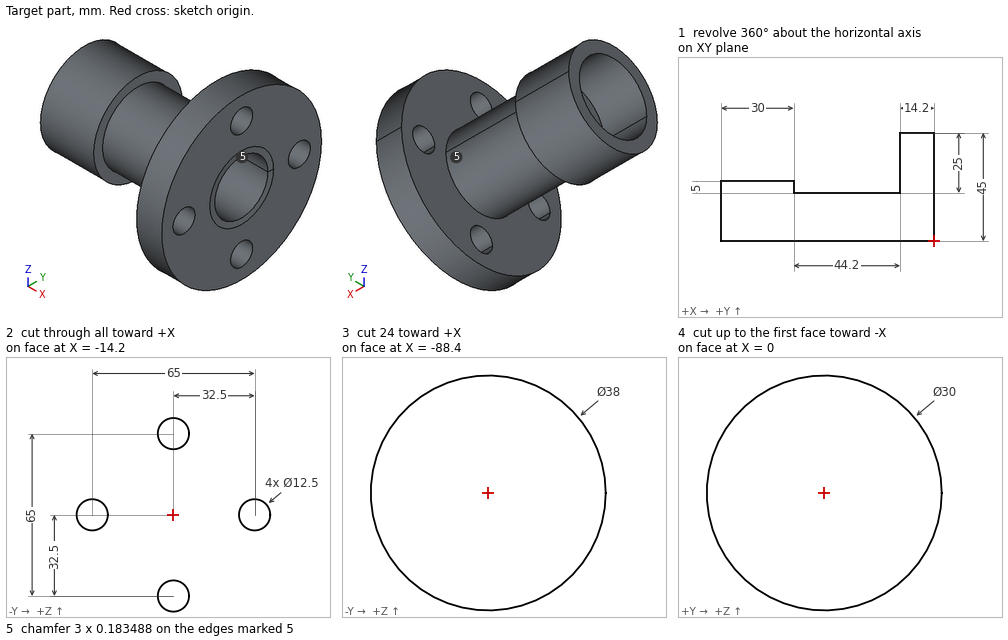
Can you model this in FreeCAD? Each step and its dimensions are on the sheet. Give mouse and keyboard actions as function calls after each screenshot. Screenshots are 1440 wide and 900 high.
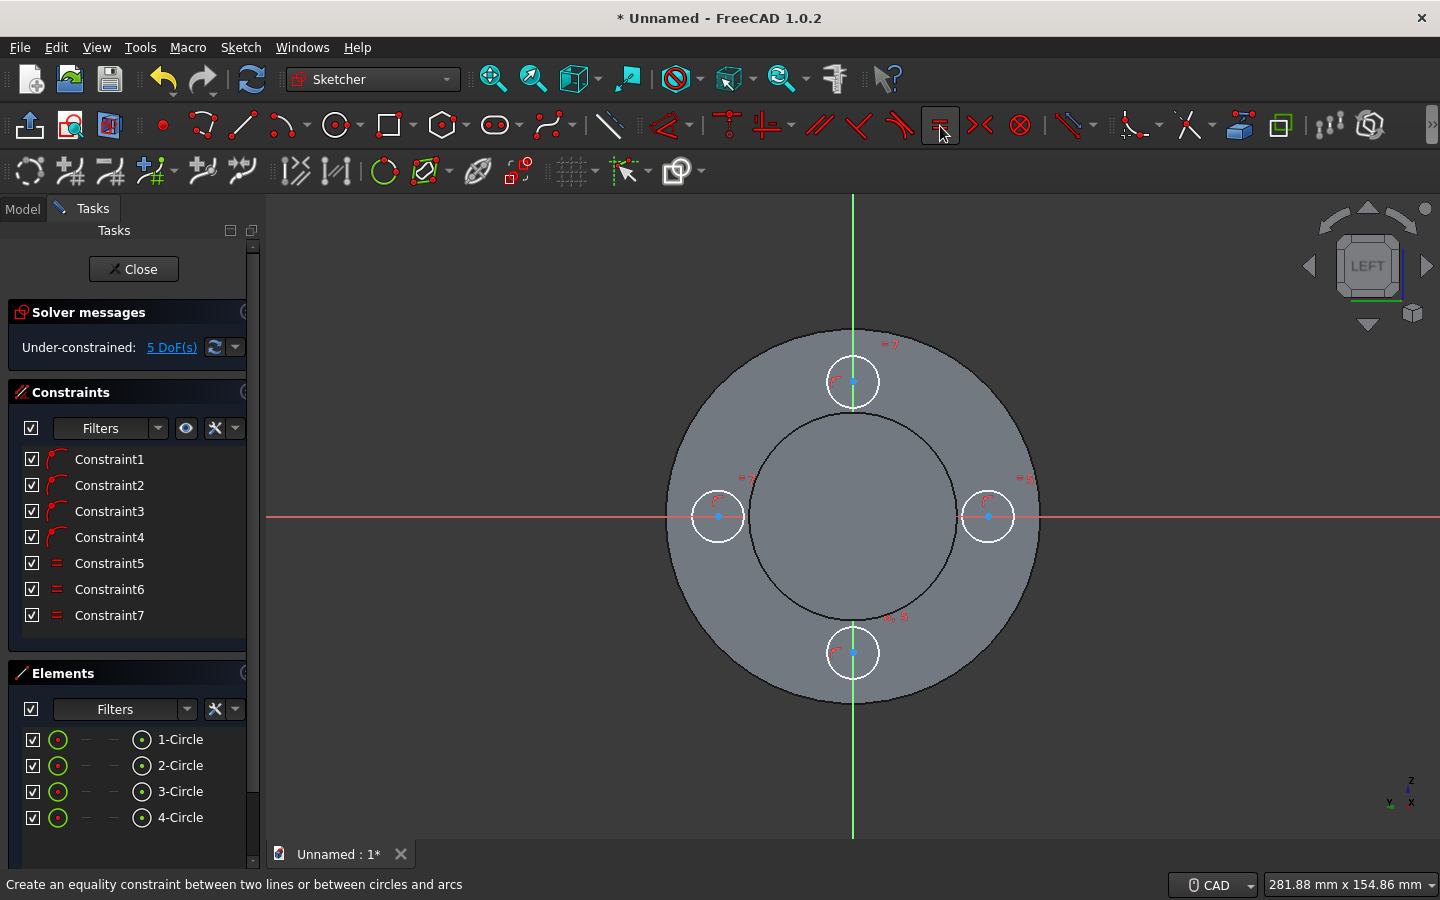
key(d)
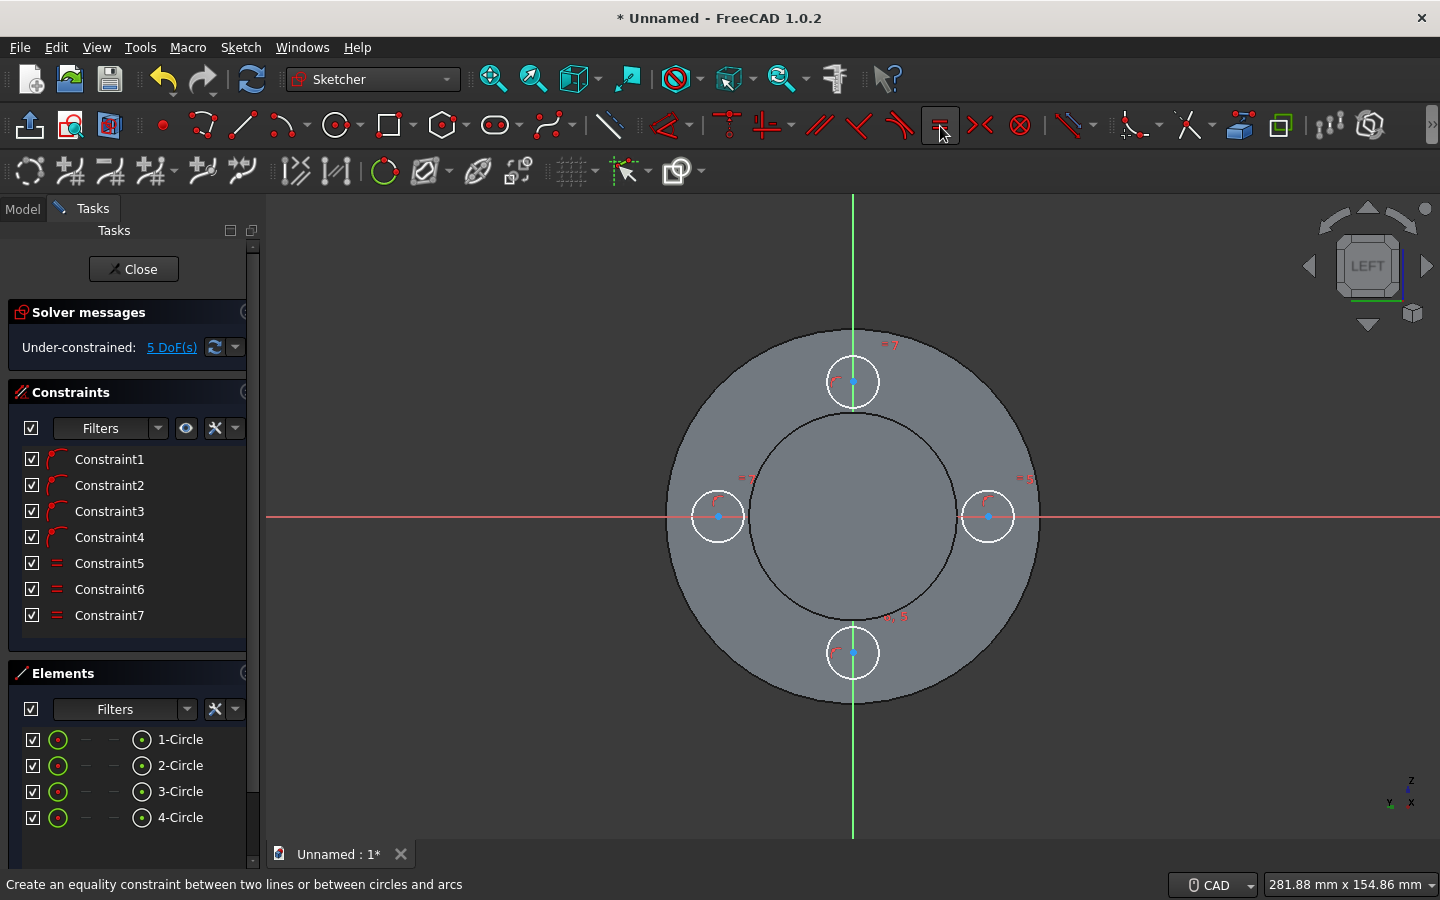
click(1006, 498)
click(1028, 475)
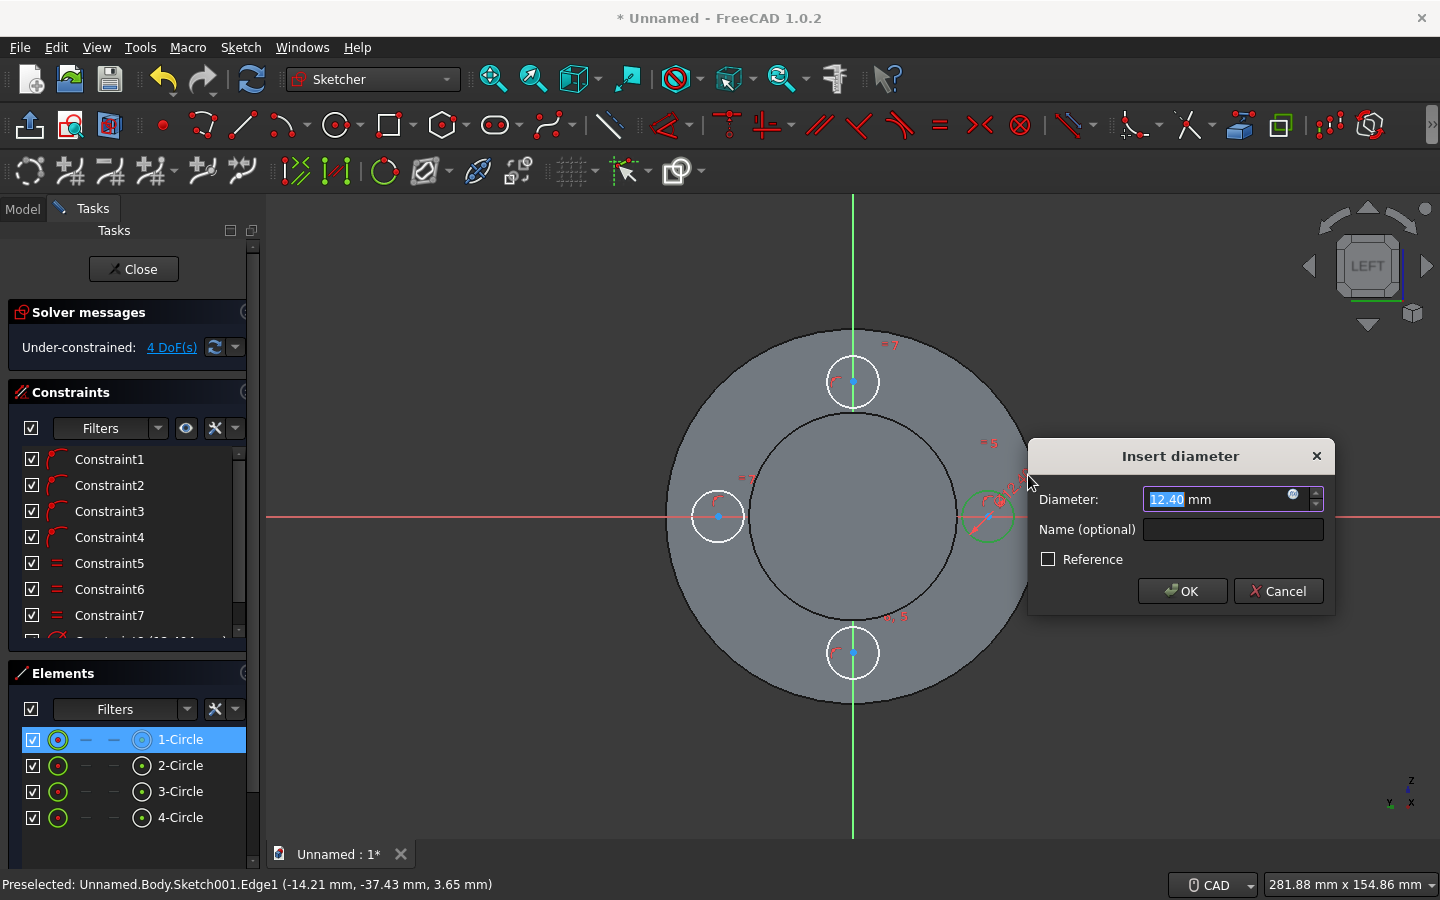
text(12.5)
key(Return)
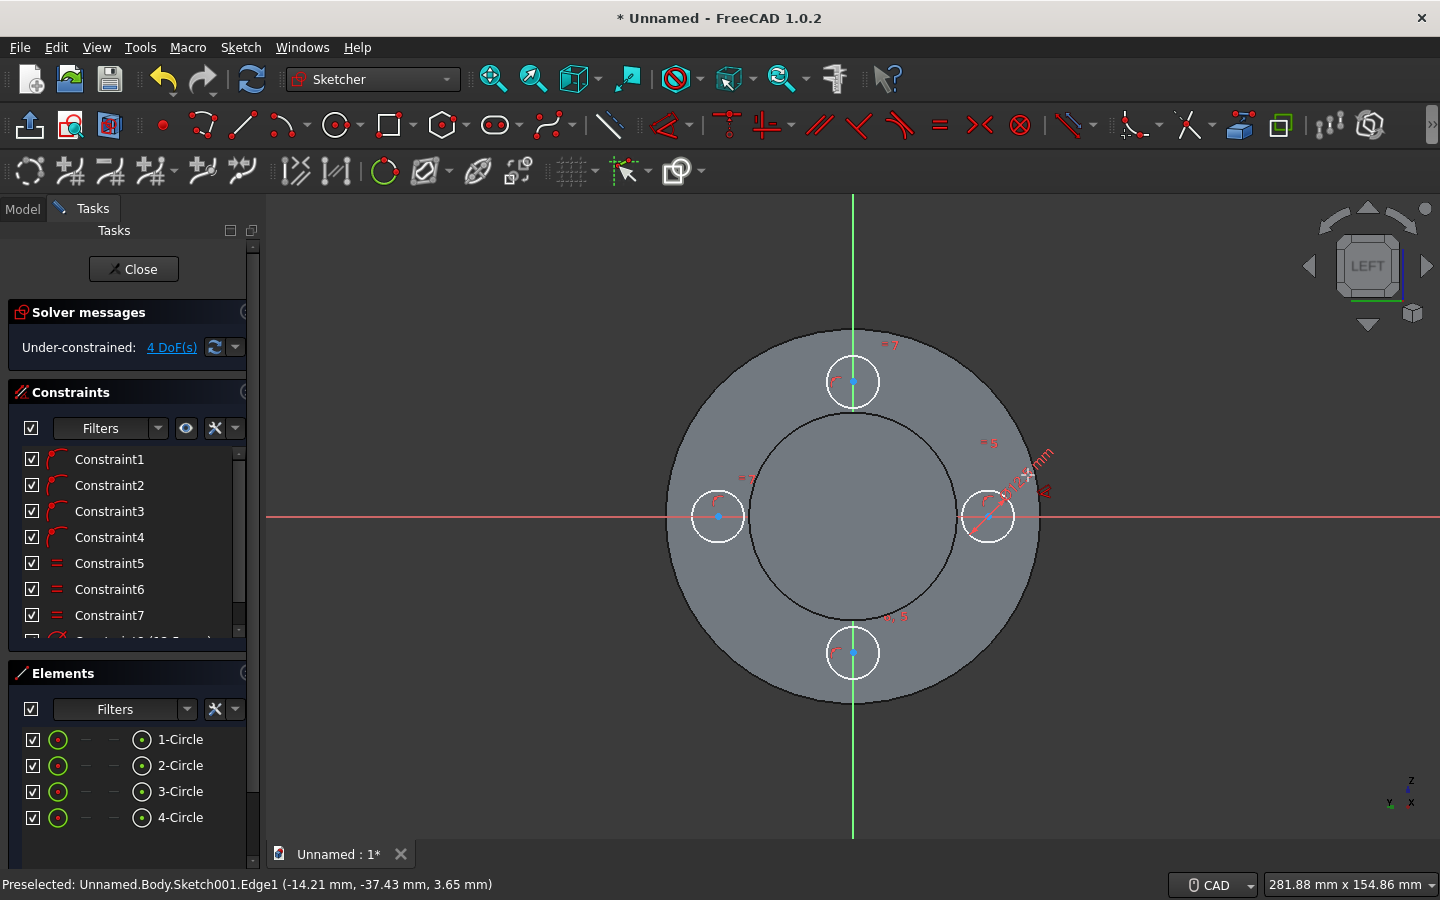
click(988, 516)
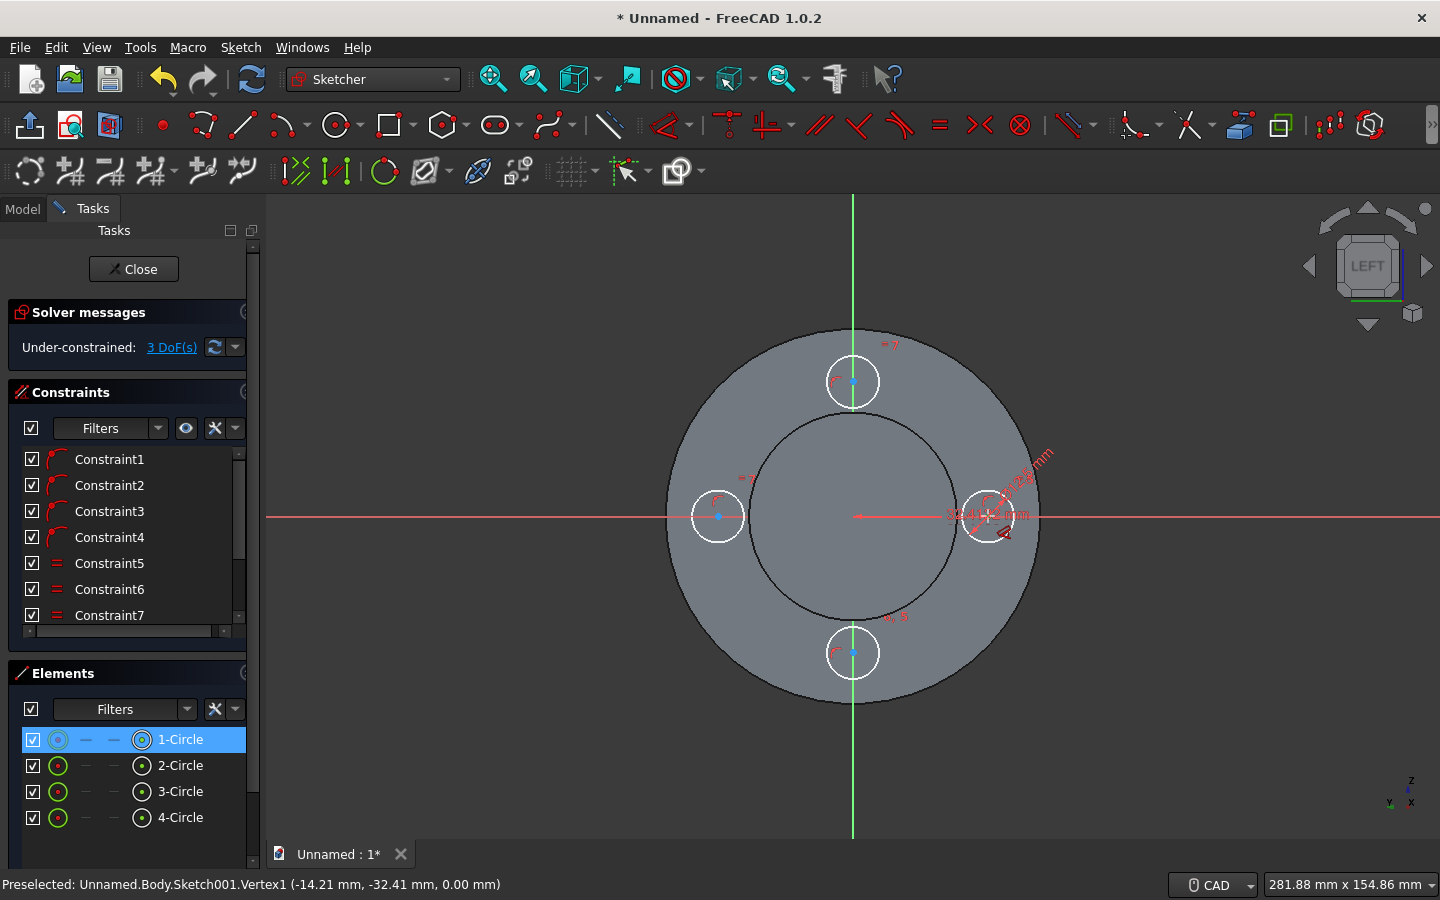
click(718, 516)
click(791, 550)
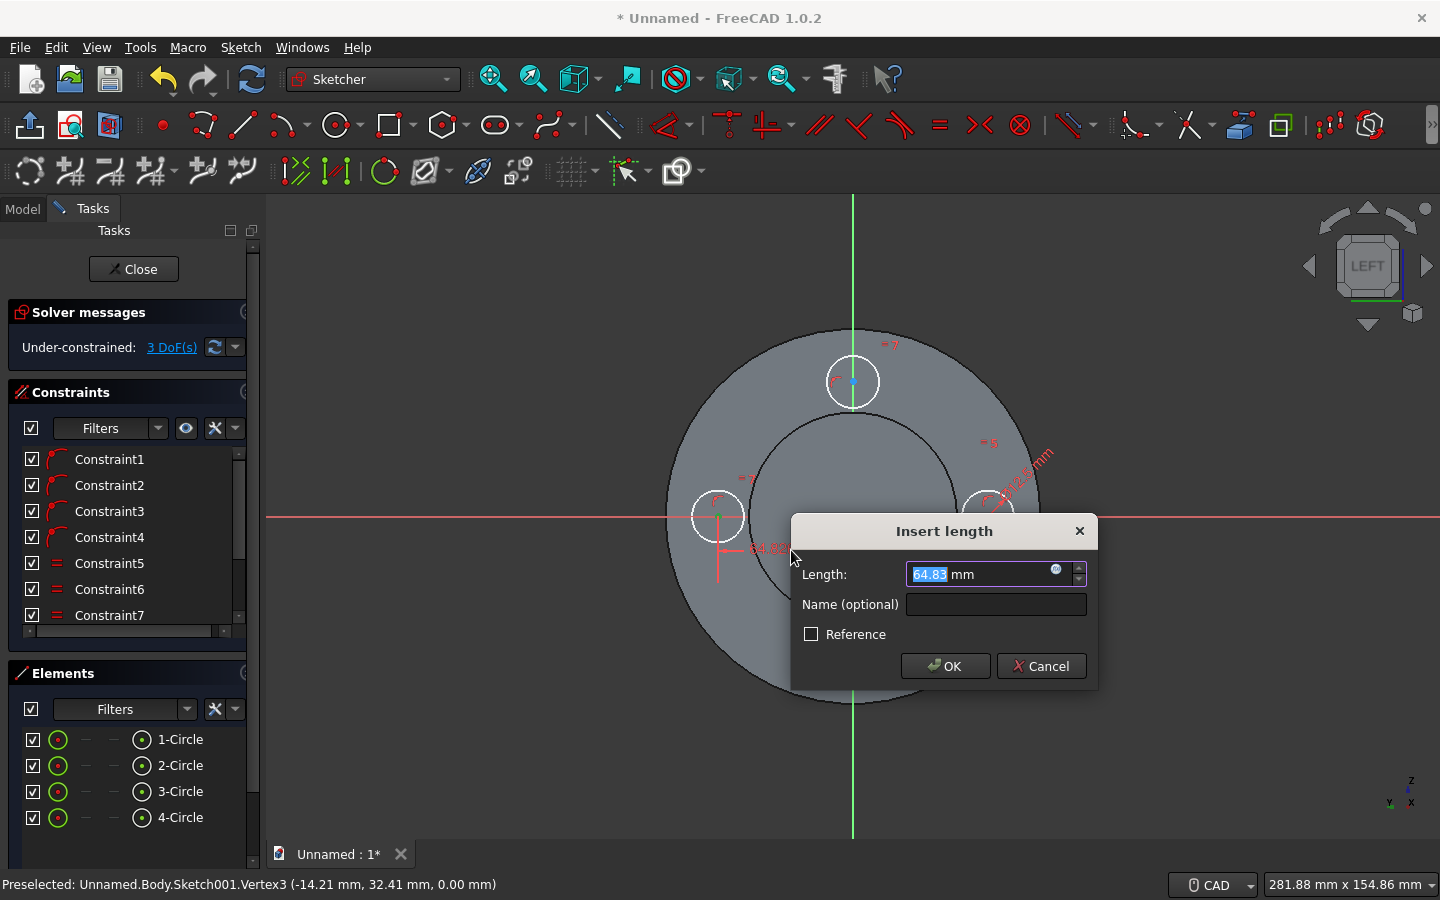
text(65)
key(Return)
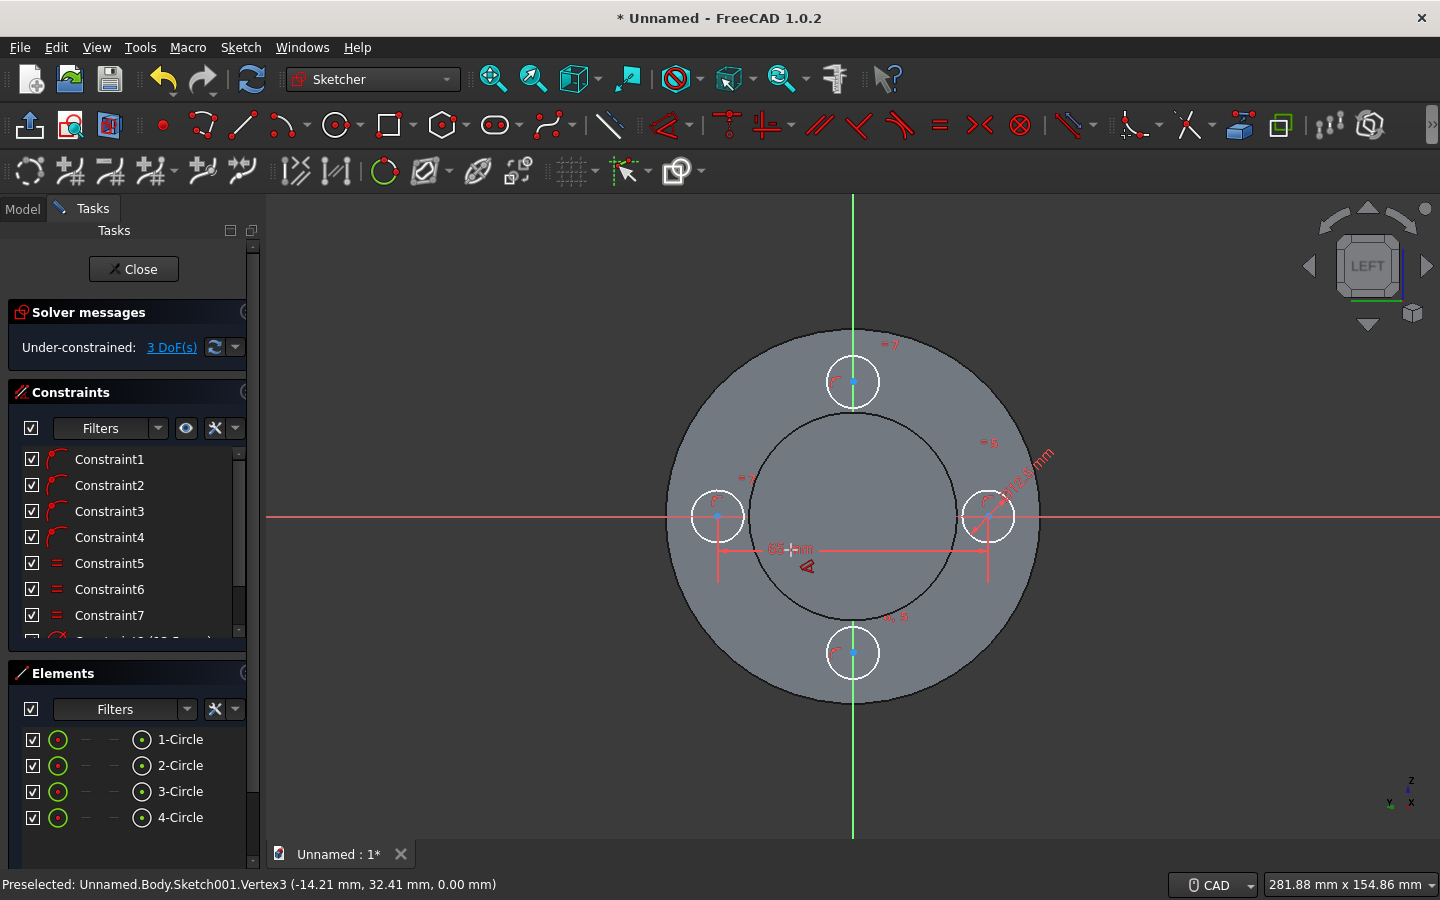
click(853, 653)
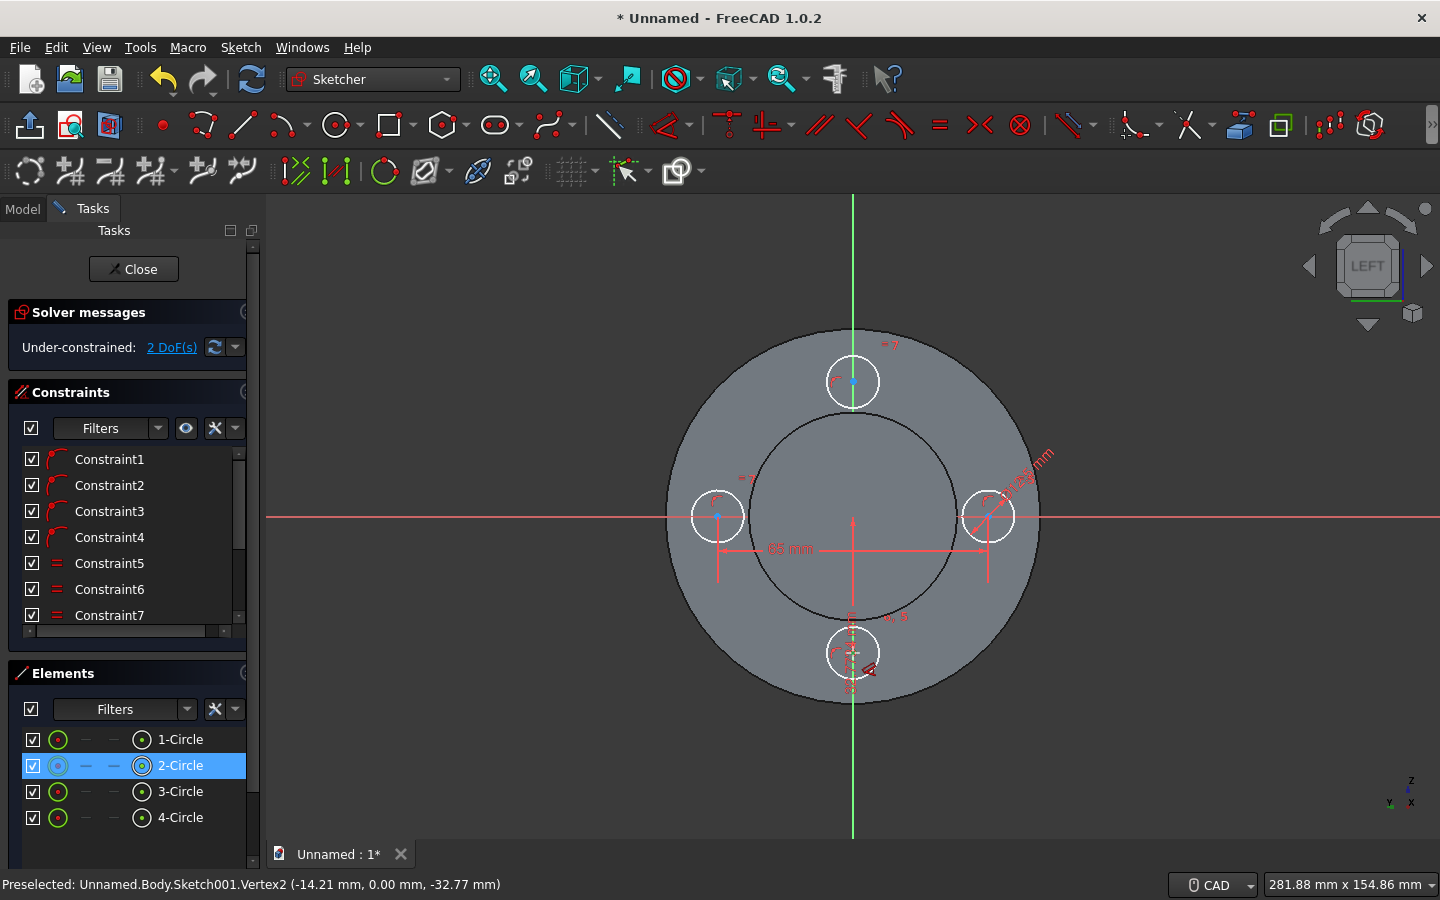
click(853, 382)
click(887, 455)